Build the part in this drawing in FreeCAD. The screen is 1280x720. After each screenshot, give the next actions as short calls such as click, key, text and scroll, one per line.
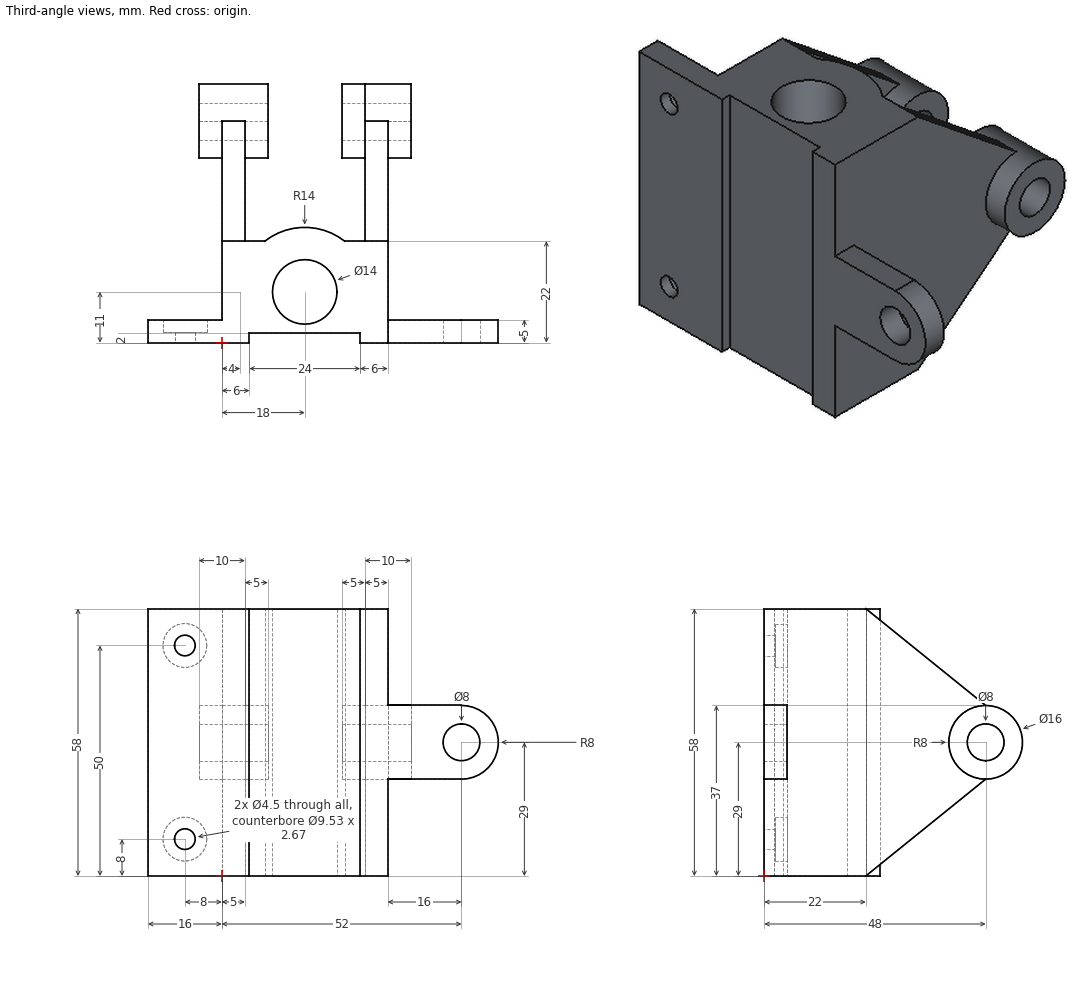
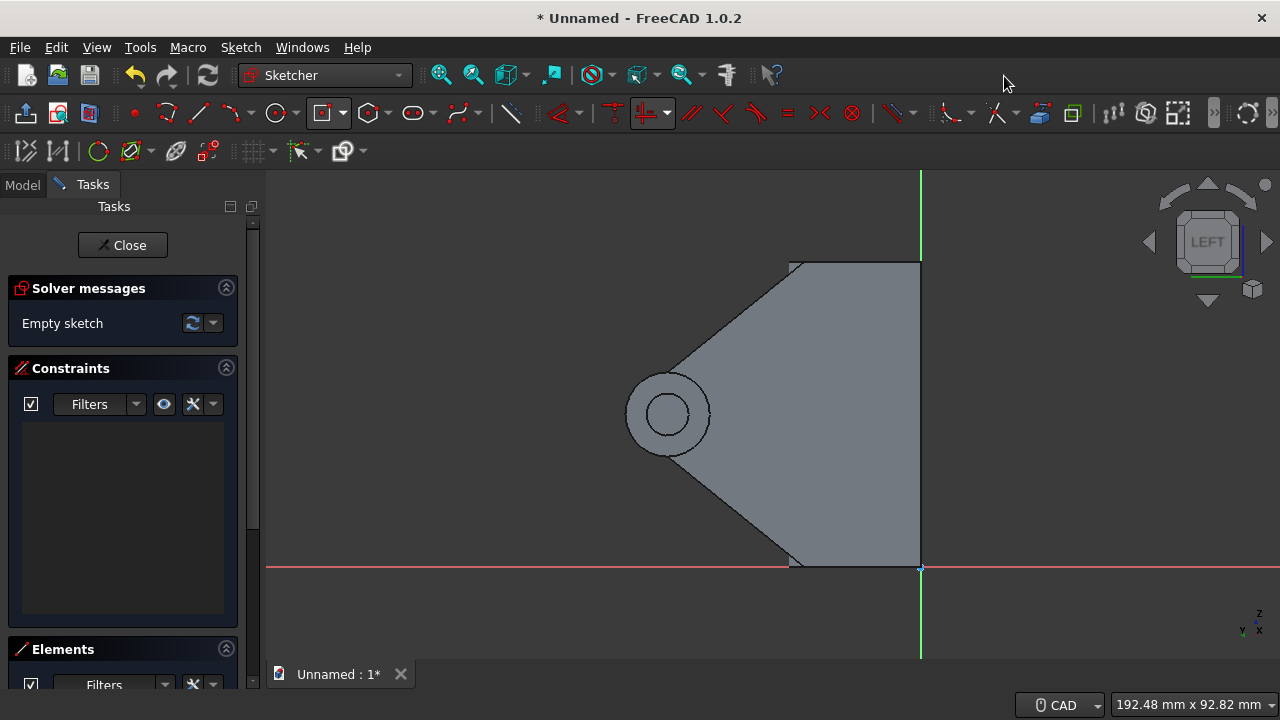
key(q)
key(s)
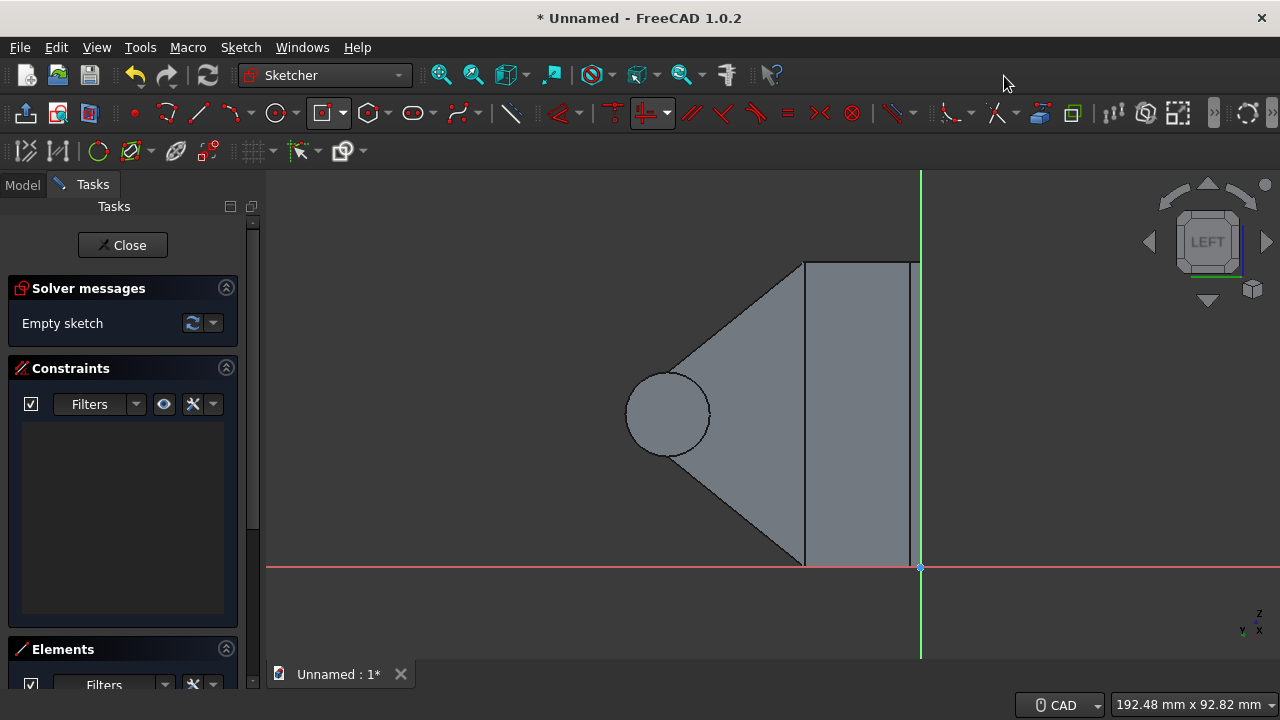
scroll(662, 414, up, 10)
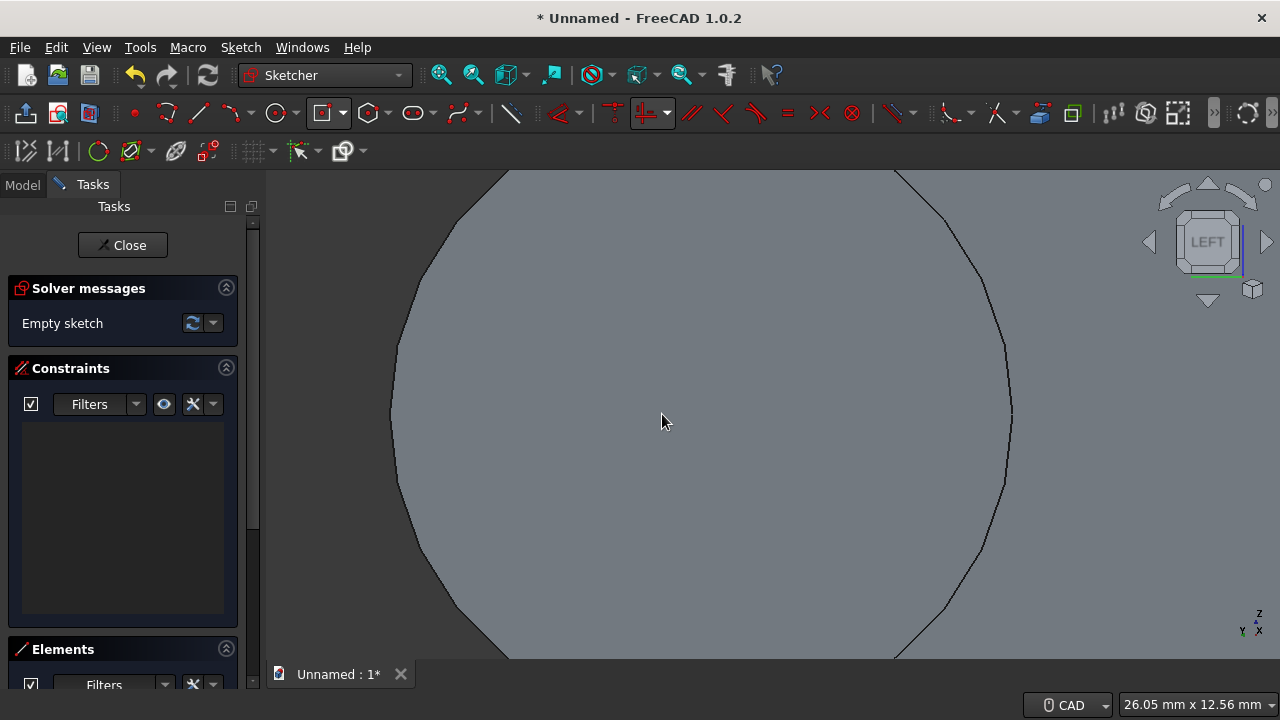
key(g)
key(c)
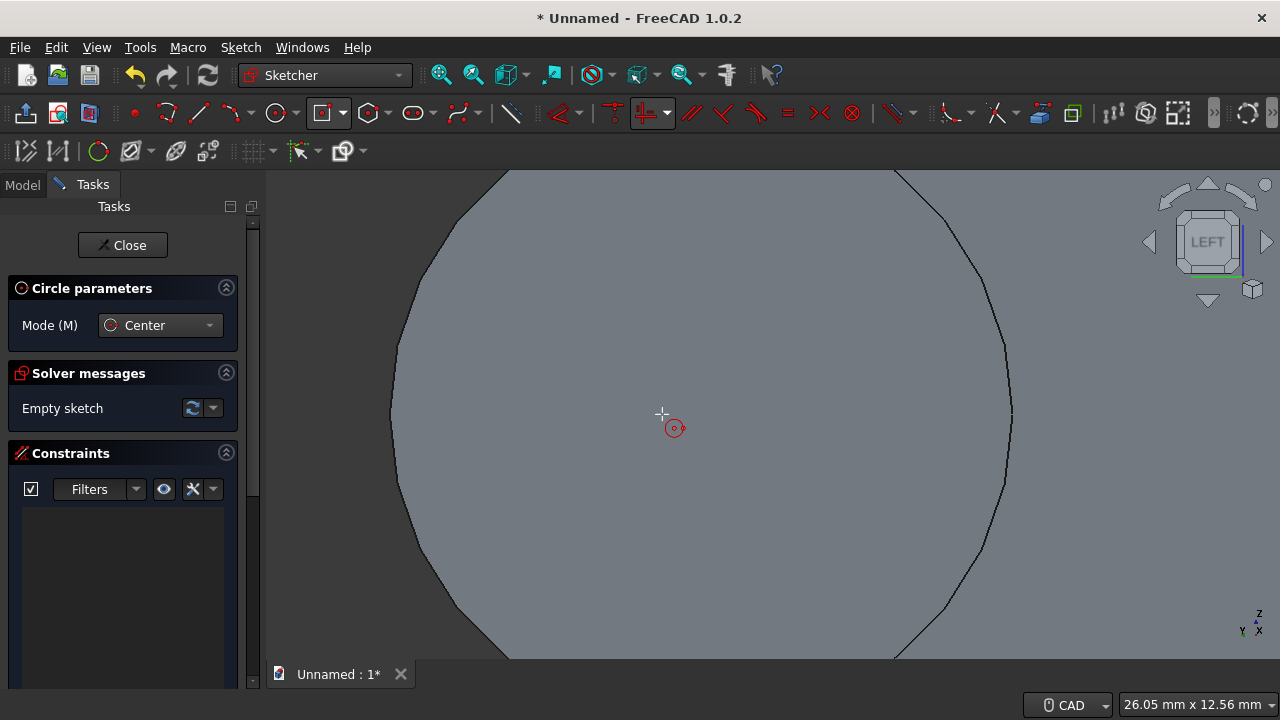
click(701, 414)
move(811, 304)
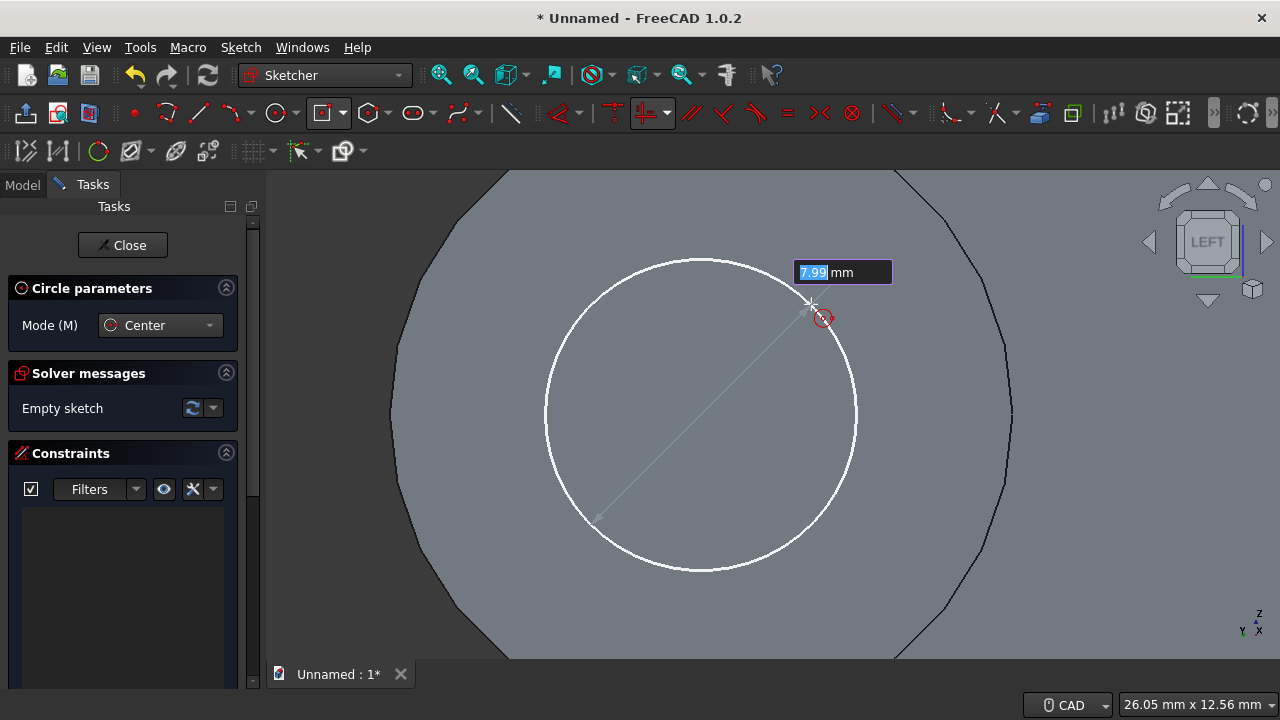
text(8)
key(Return)
key(Escape)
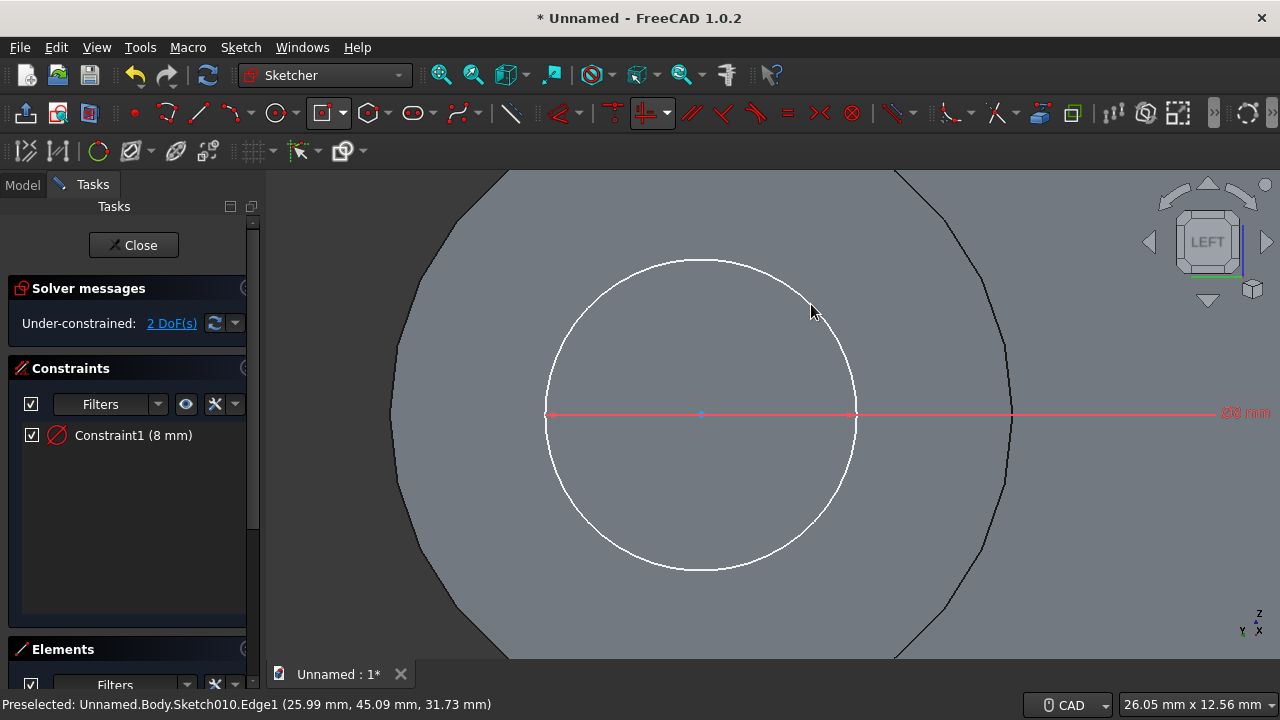
key(d)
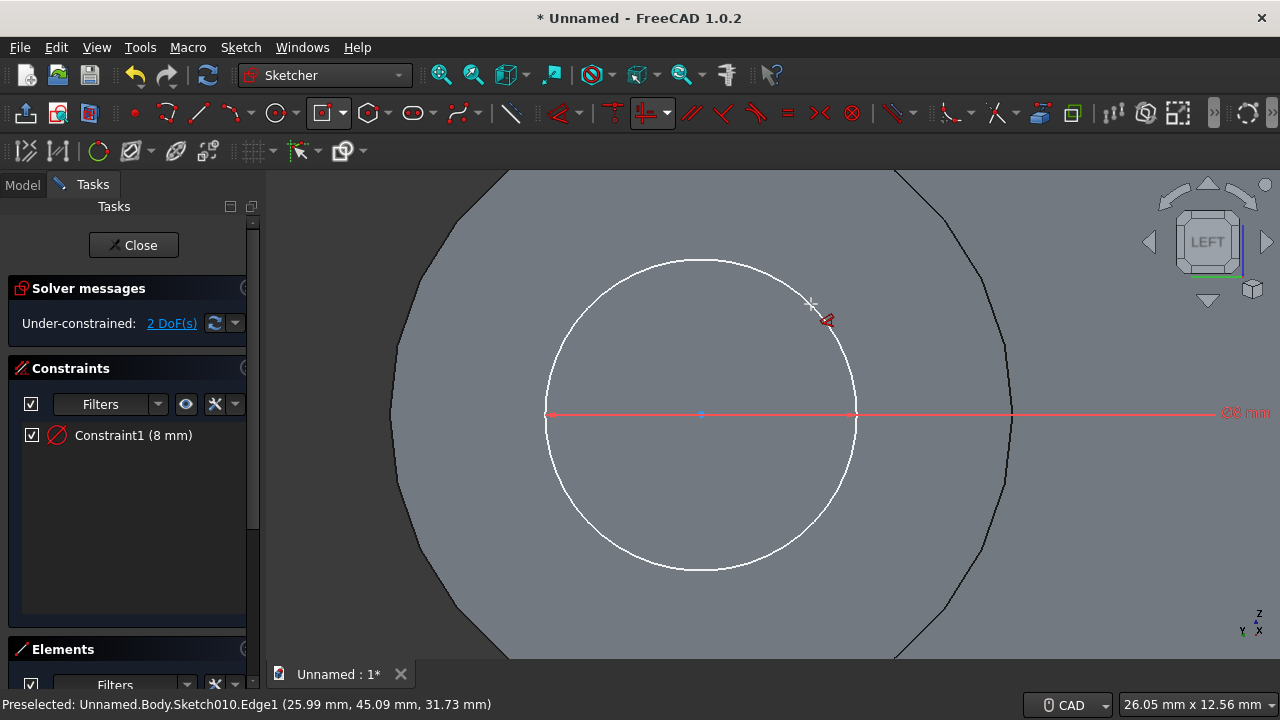
click(701, 415)
click(908, 381)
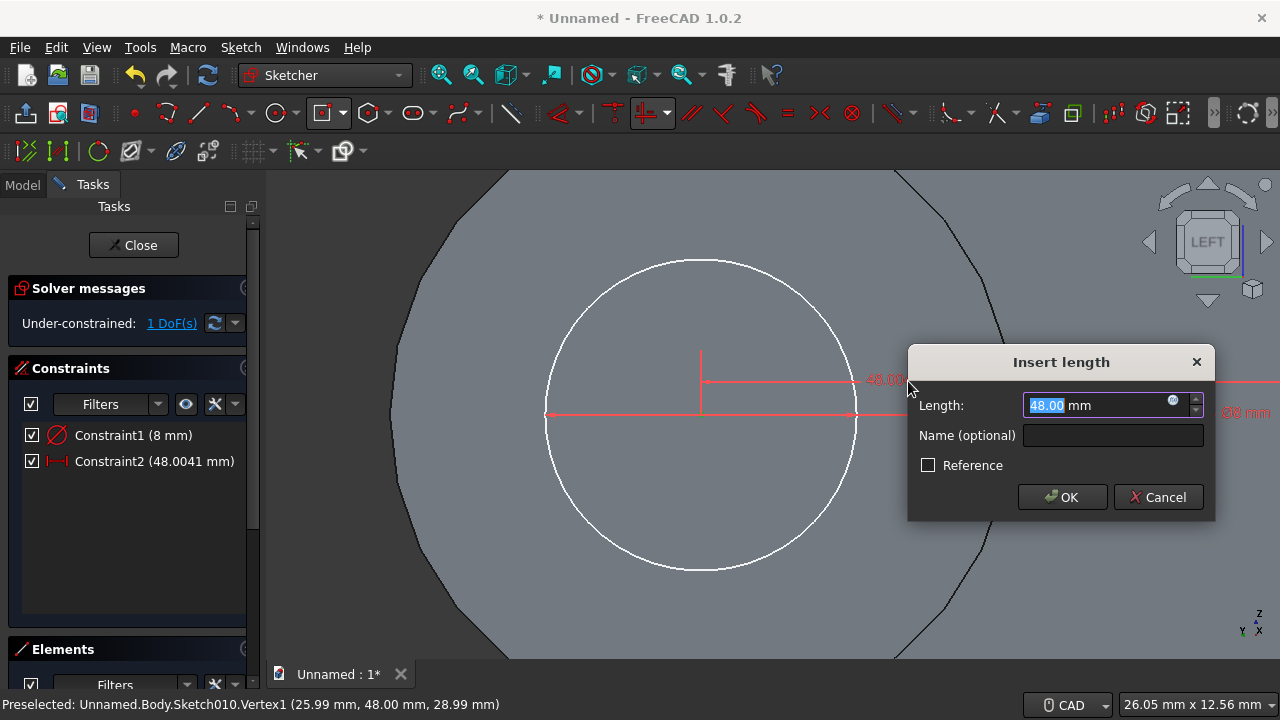
text(48)
key(Return)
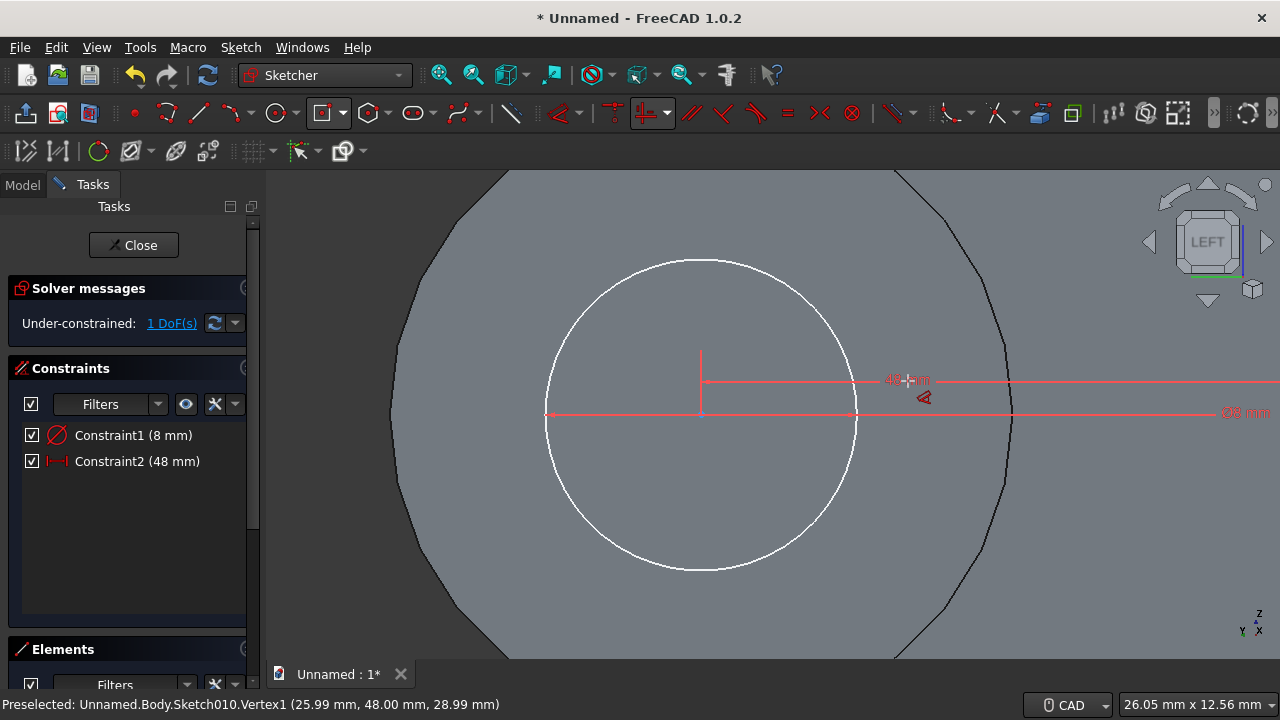
click(701, 415)
click(667, 523)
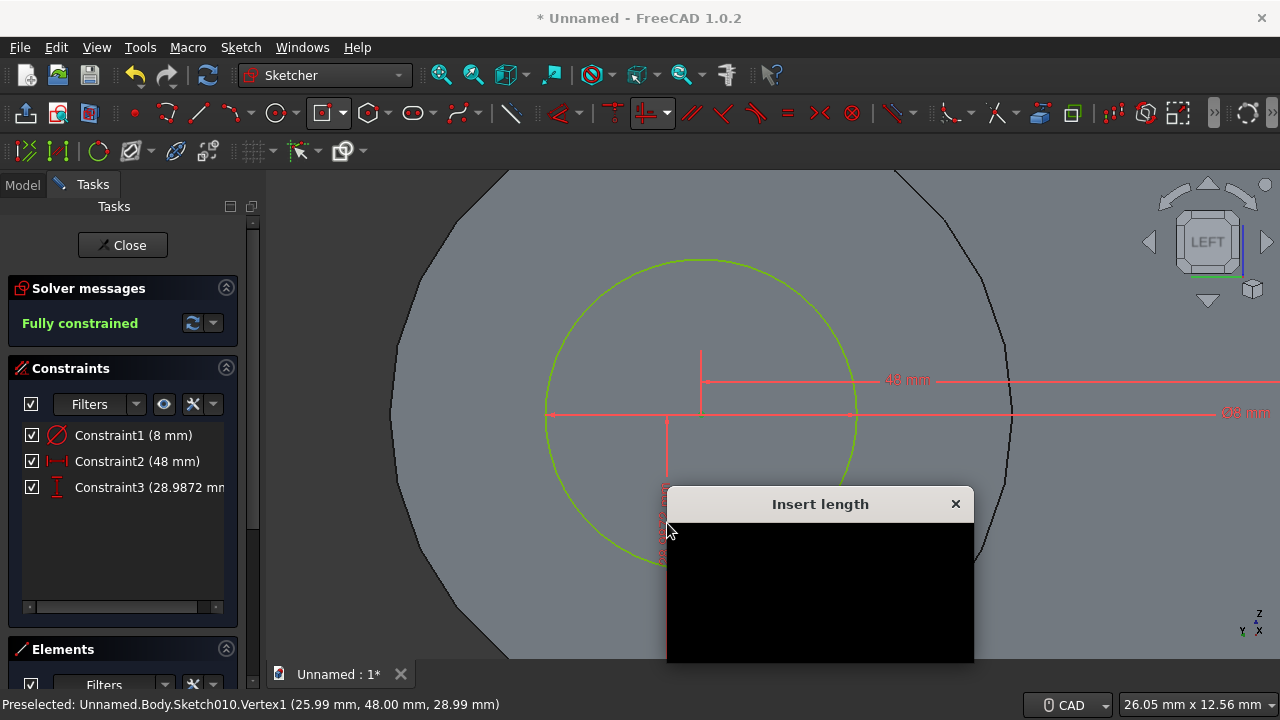
text(29)
key(Return)
key(Escape)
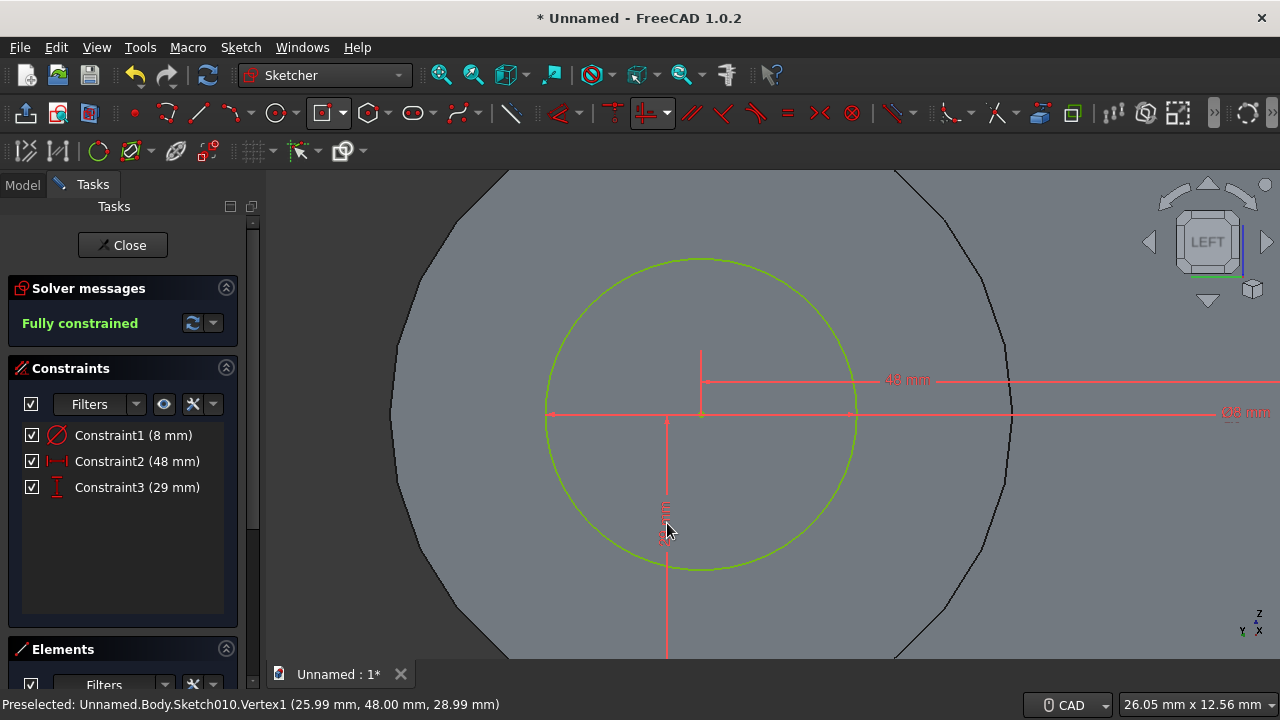
click(123, 245)